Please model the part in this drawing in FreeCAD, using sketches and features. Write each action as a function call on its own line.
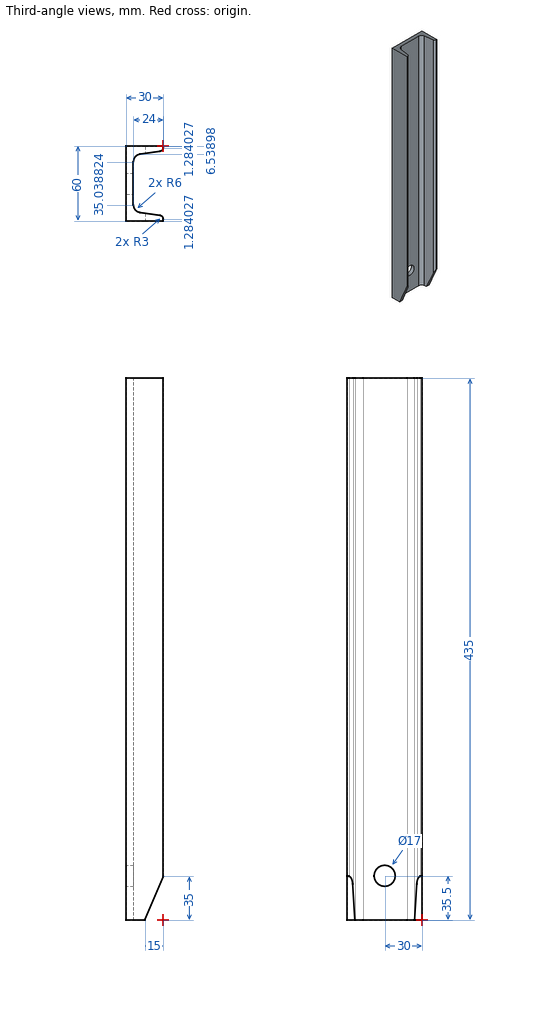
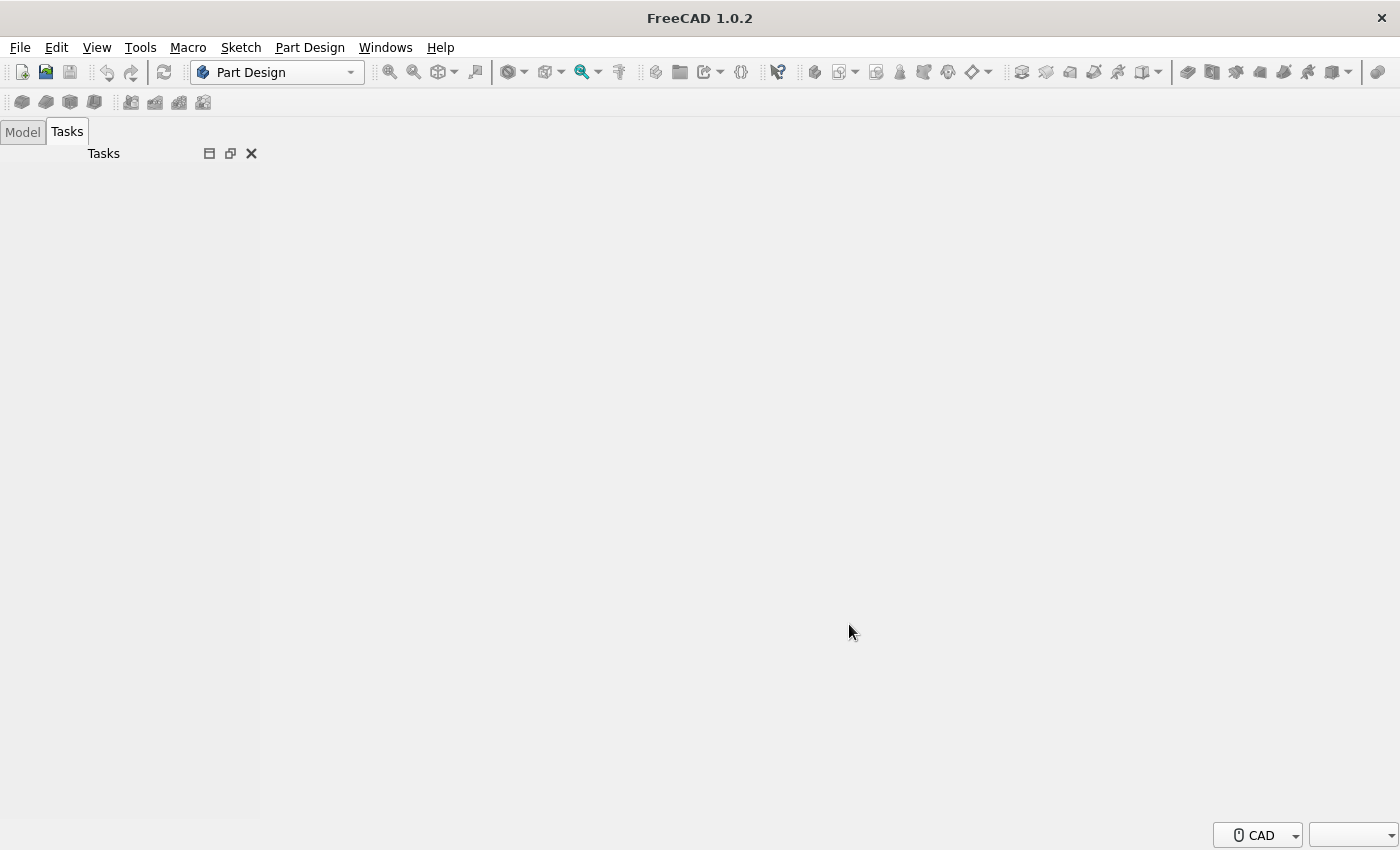
click(22, 72)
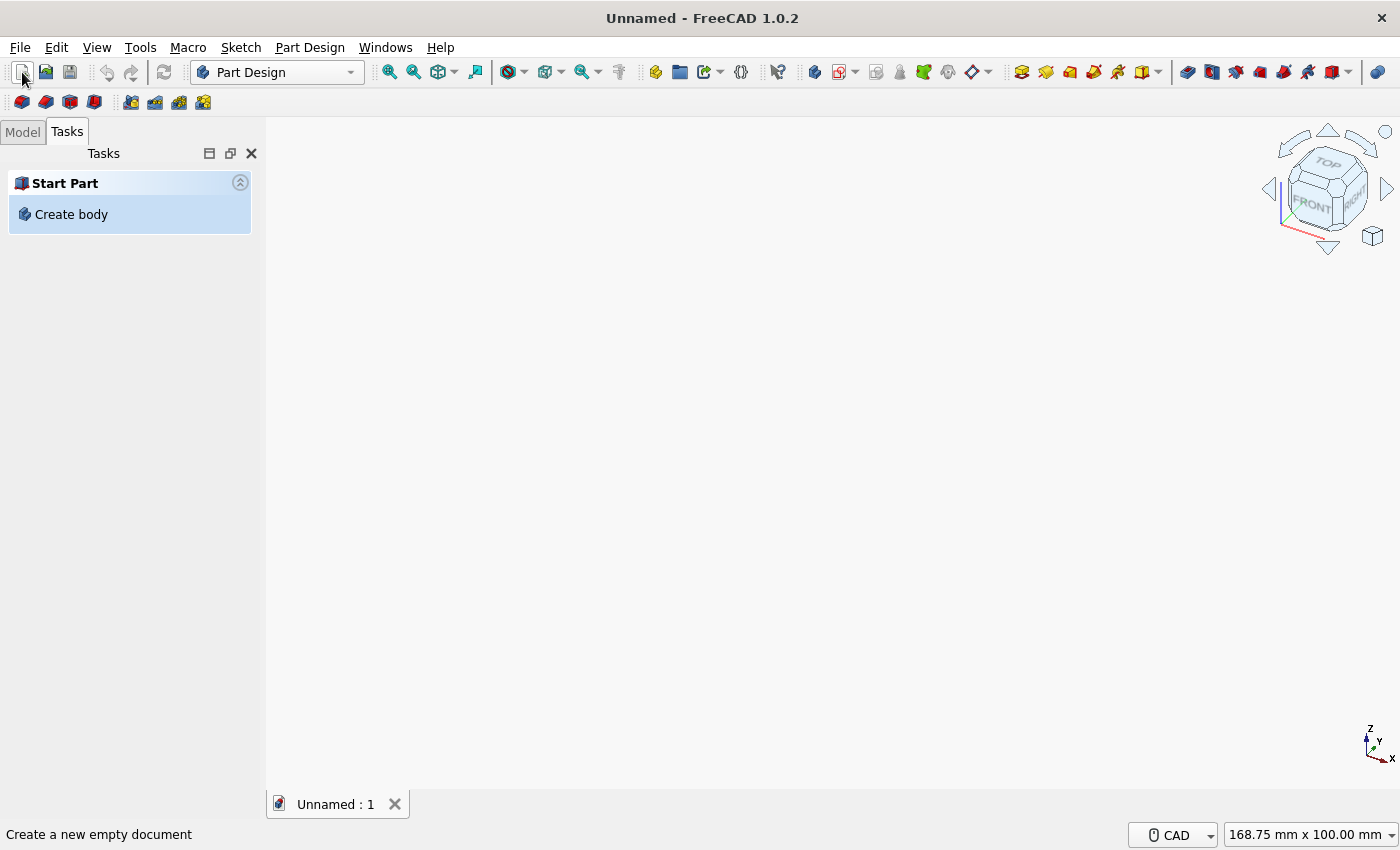
click(840, 72)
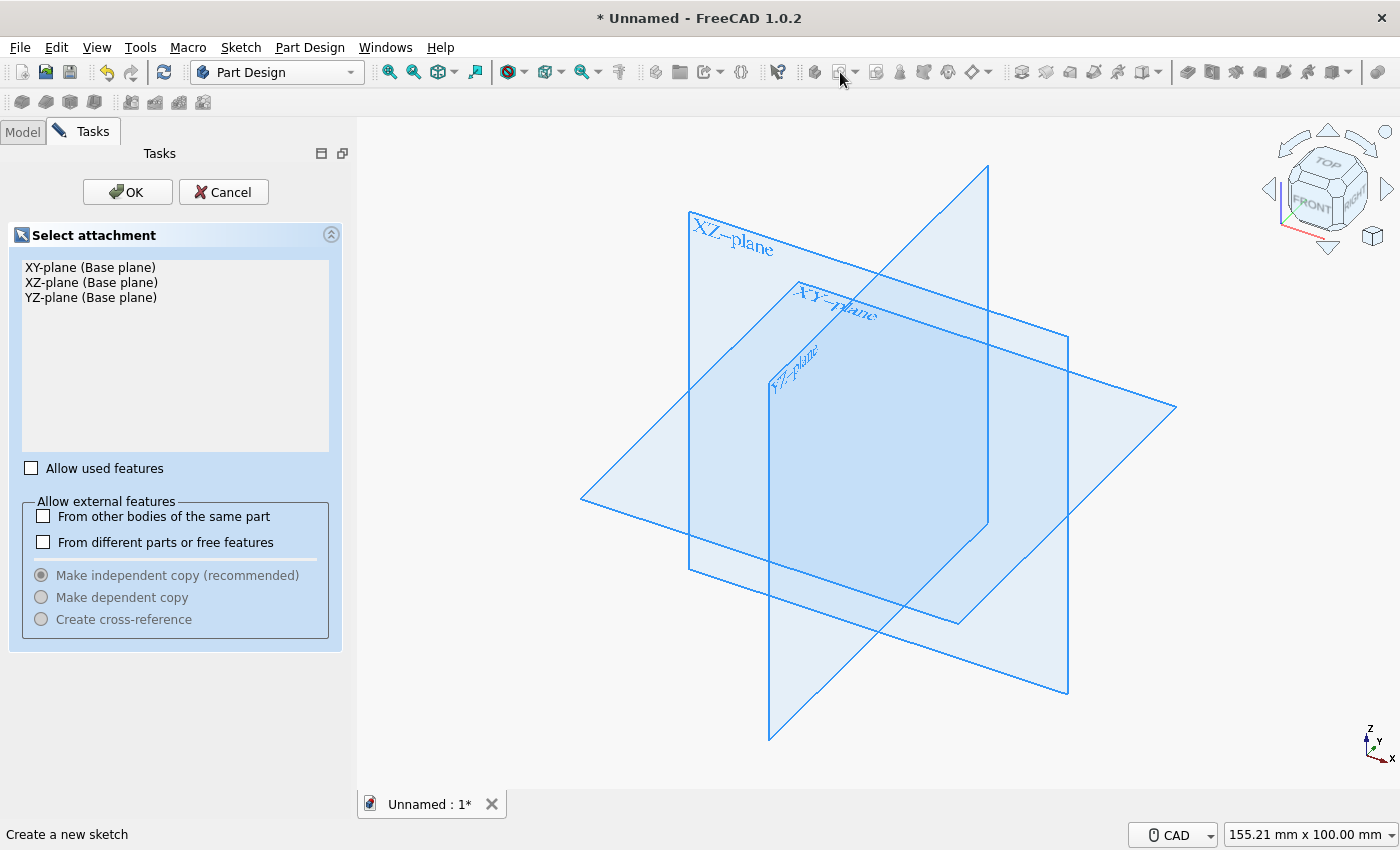
click(82, 268)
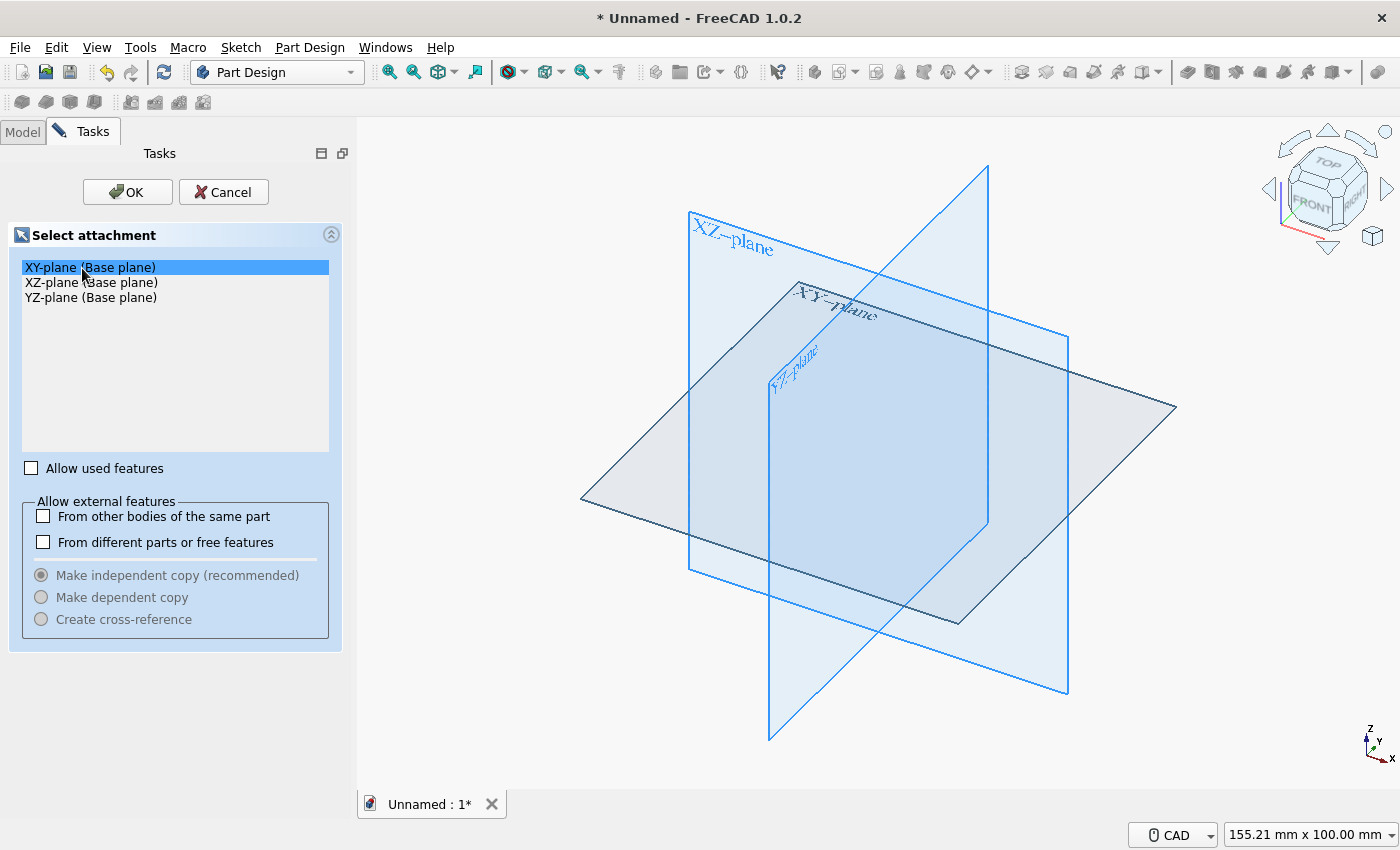
click(128, 192)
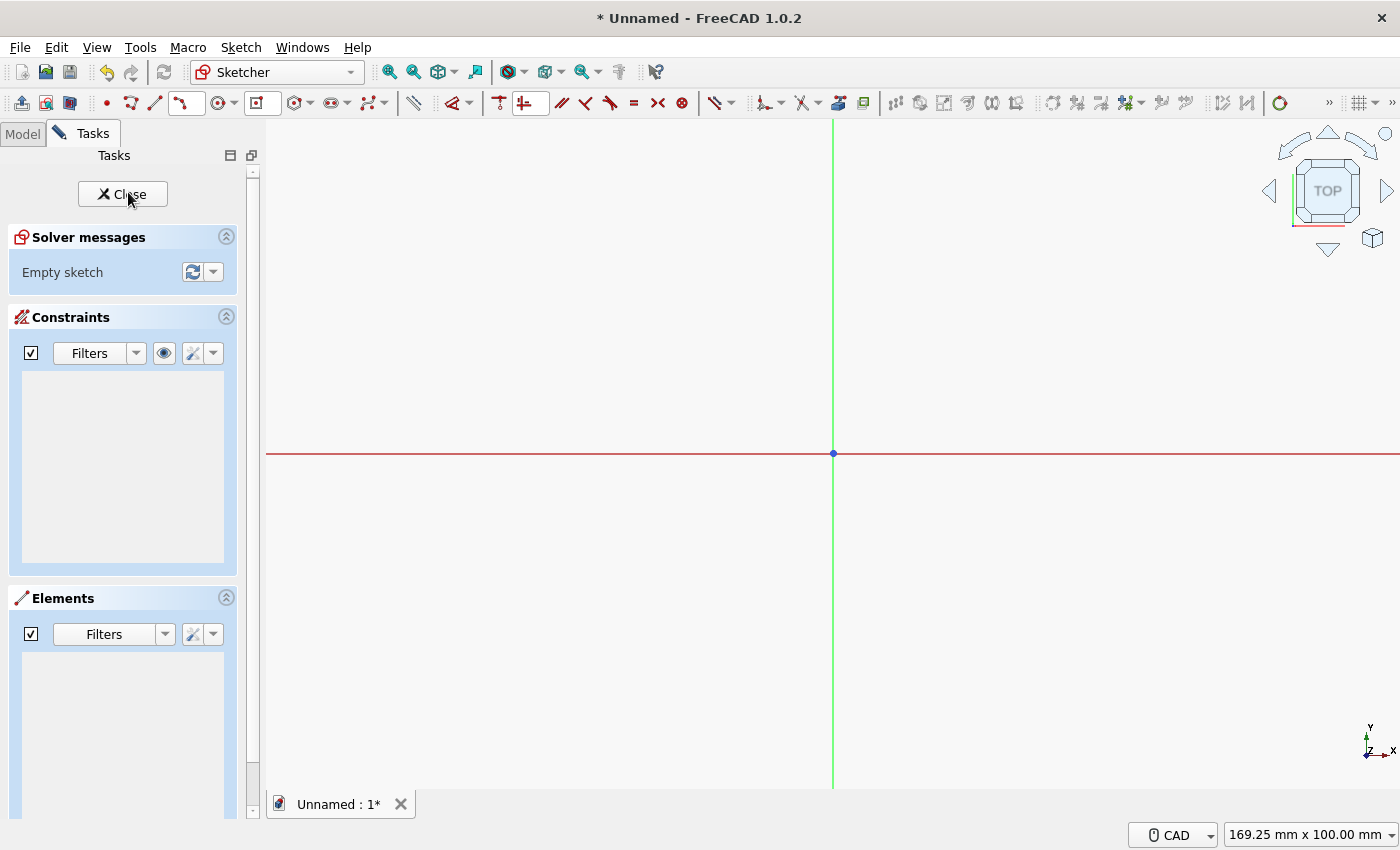
scroll(909, 147, down, 1)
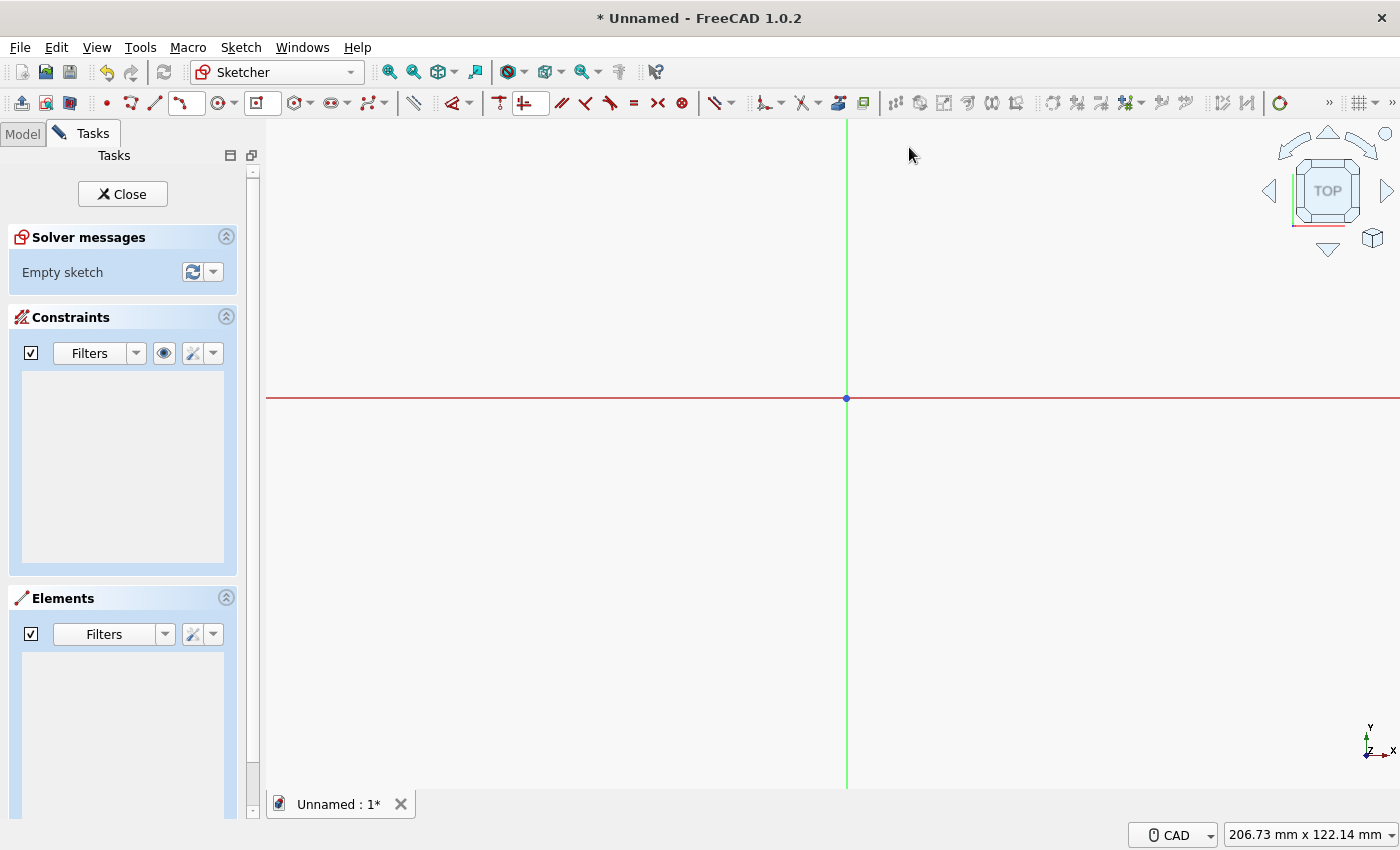
click(156, 104)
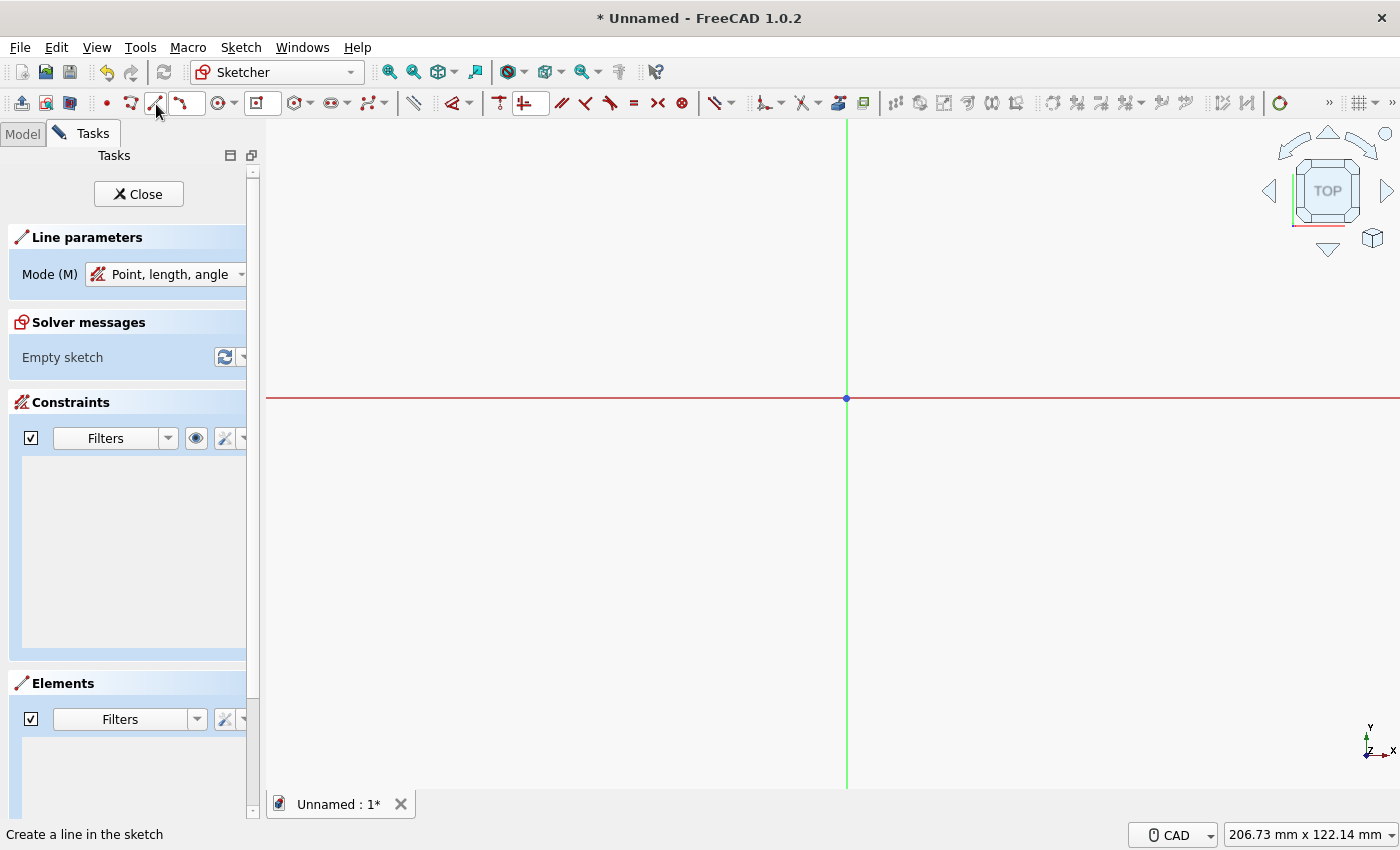
click(833, 704)
click(744, 692)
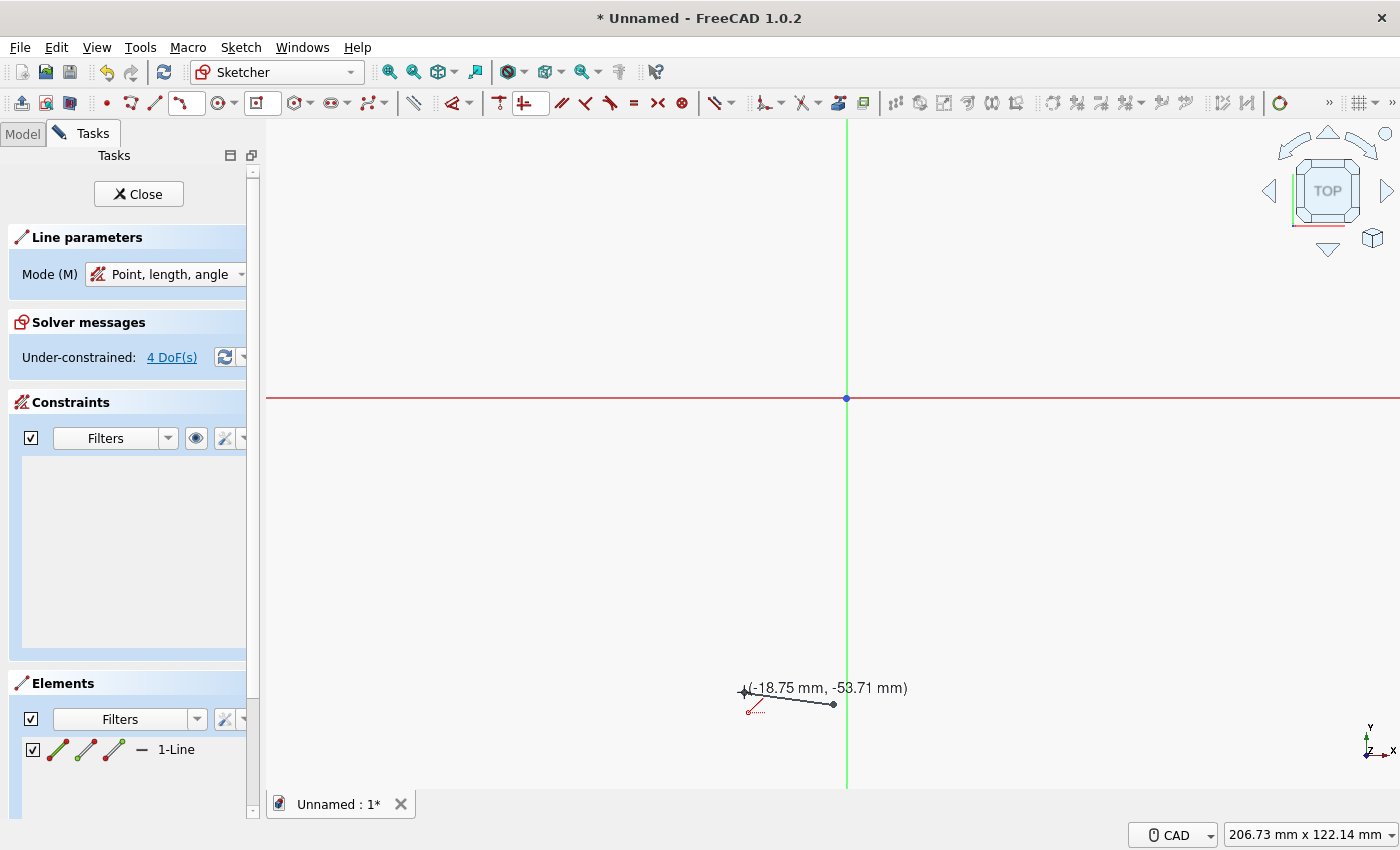
click(715, 659)
click(715, 467)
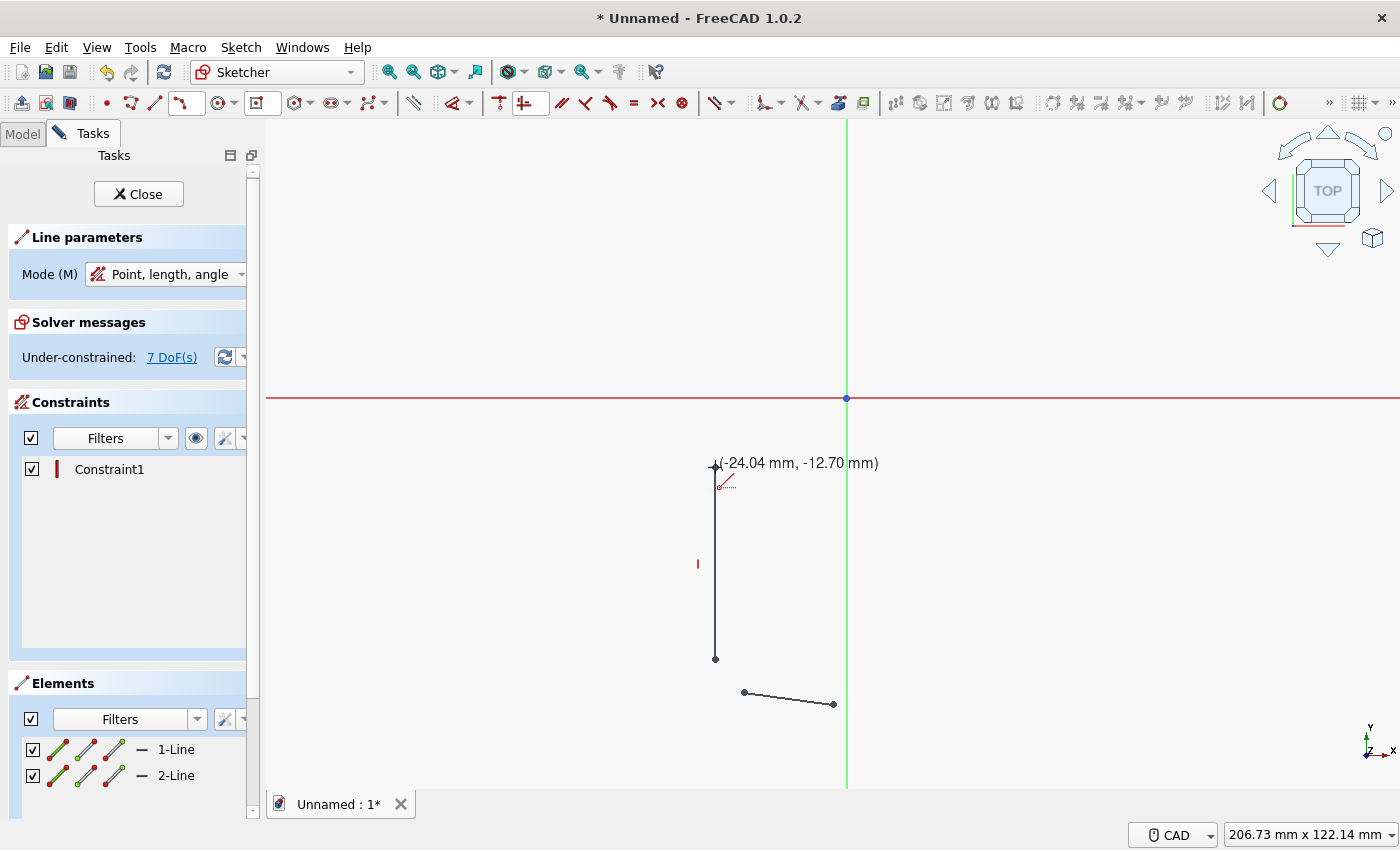
click(744, 434)
click(833, 422)